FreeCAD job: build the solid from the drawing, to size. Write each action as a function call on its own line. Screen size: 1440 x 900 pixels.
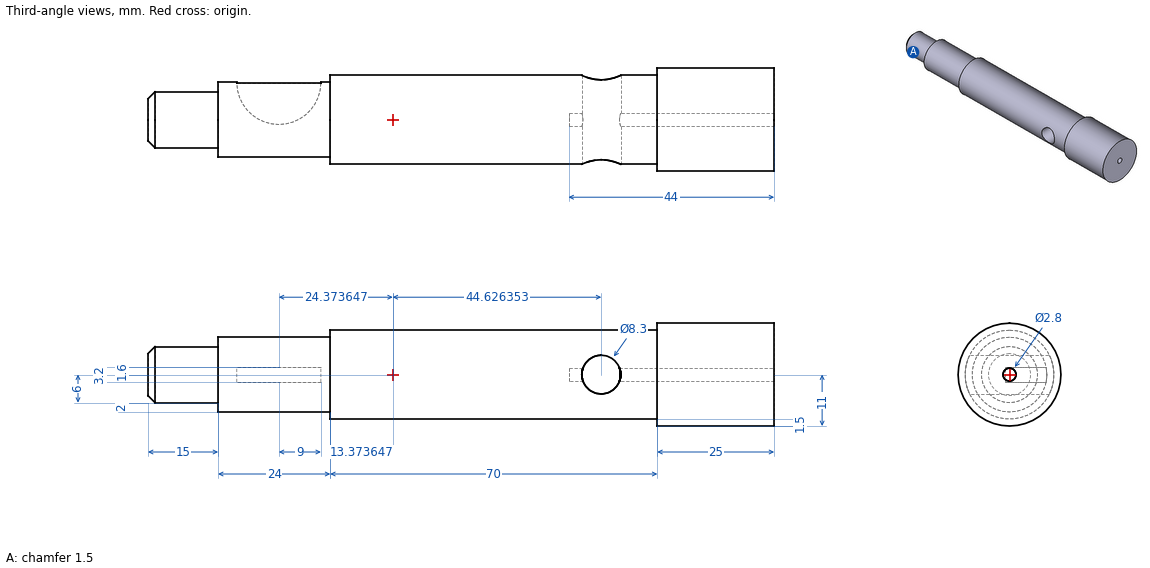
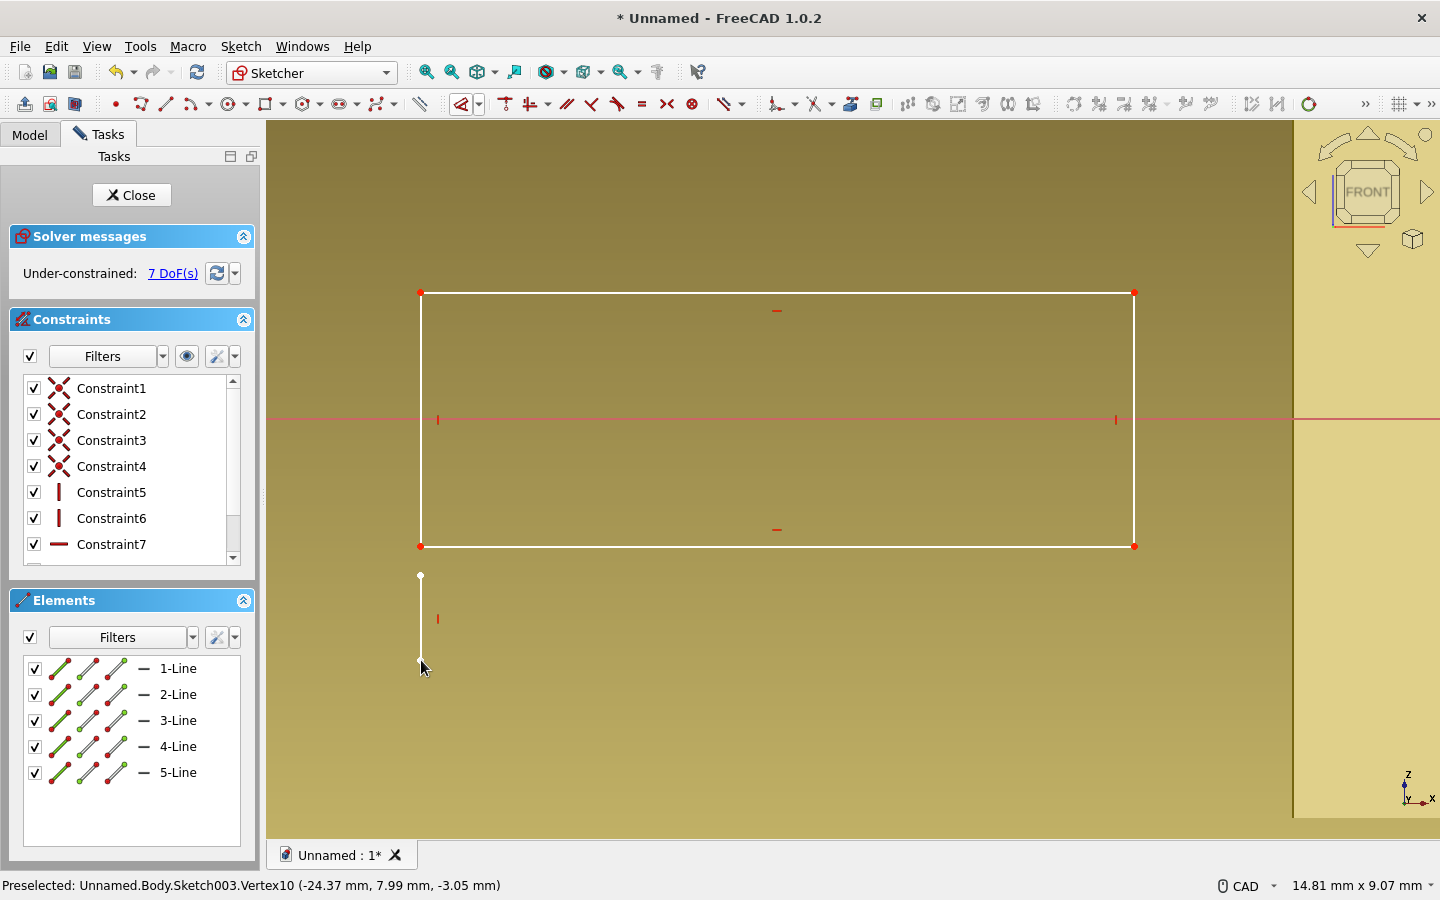
click(421, 601)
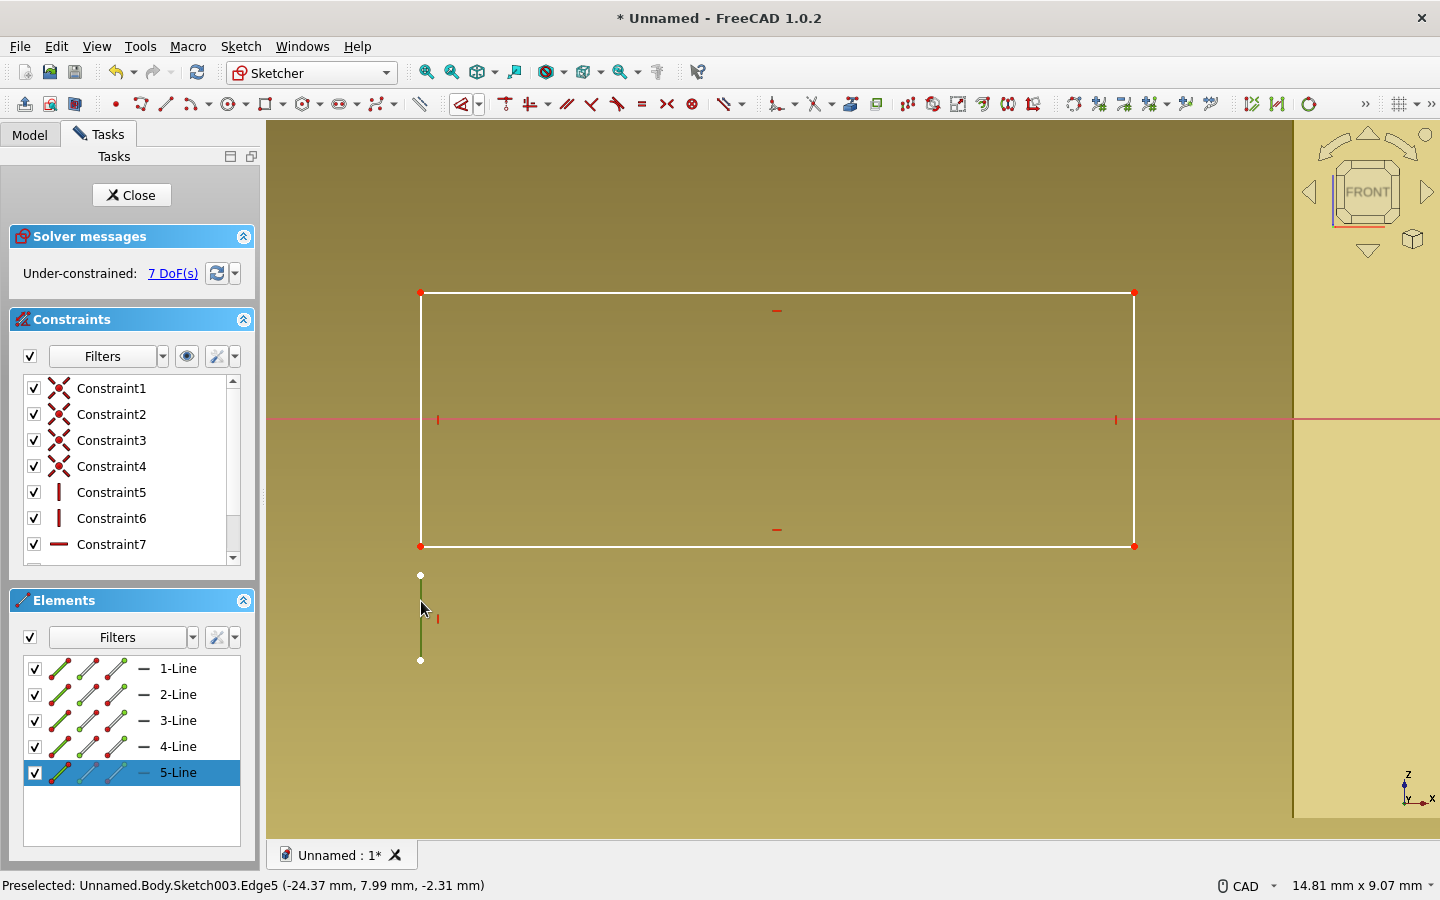
click(420, 104)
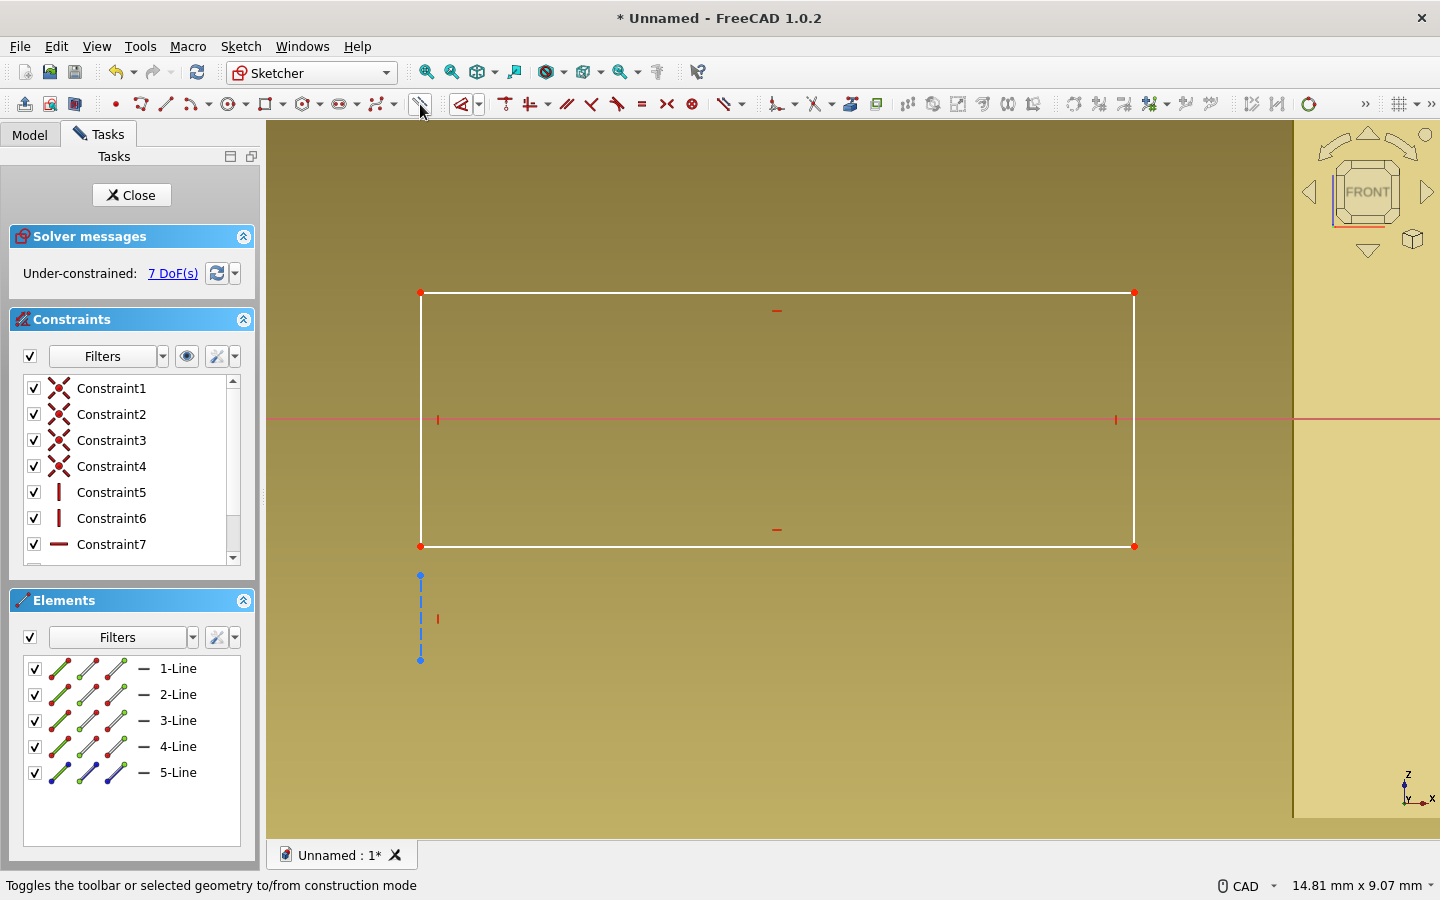
click(635, 547)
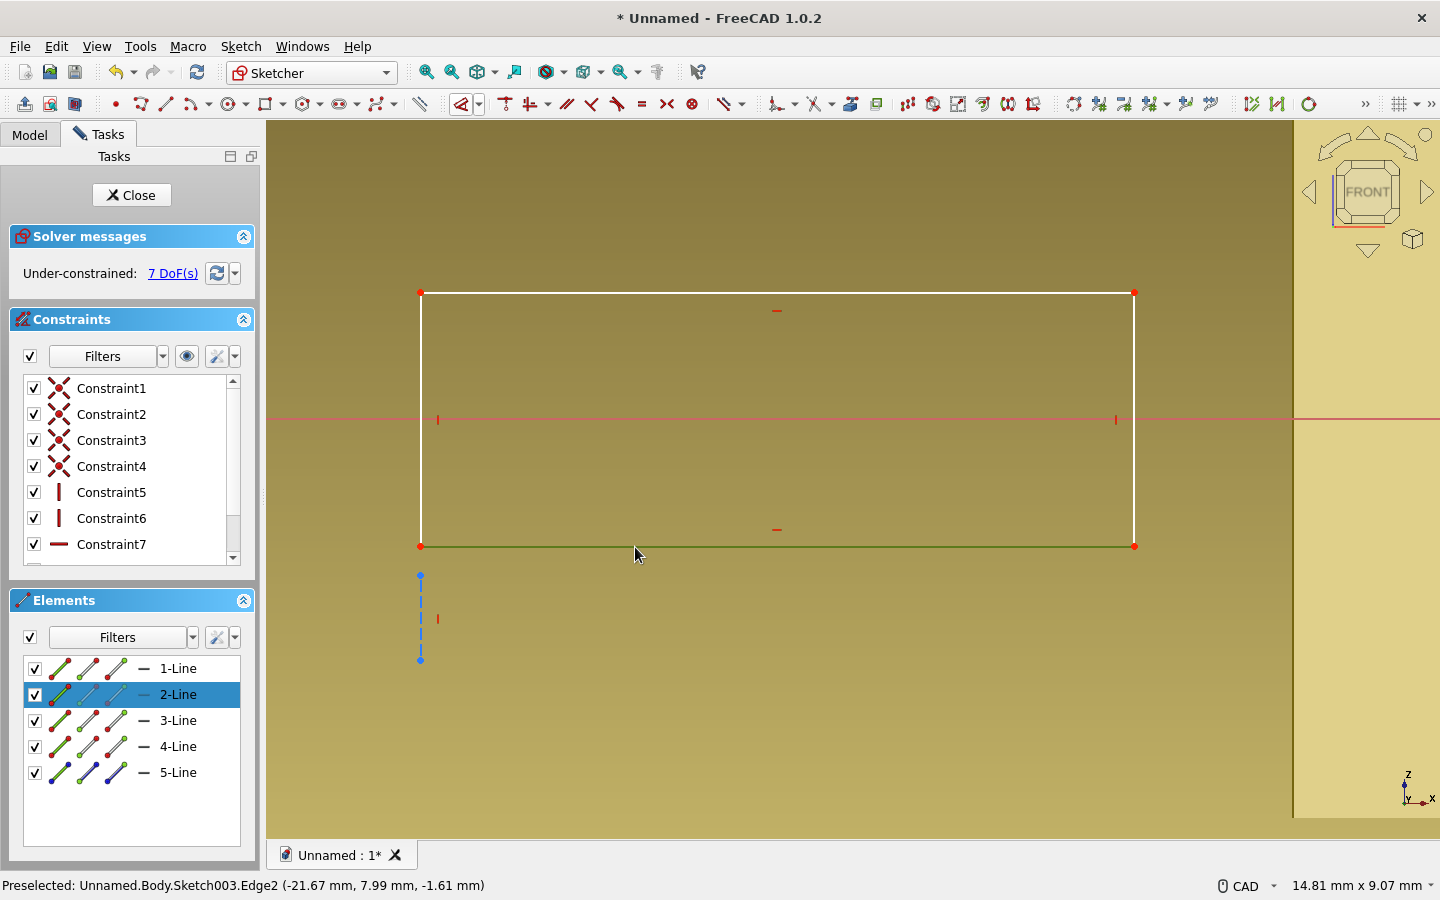
key(l)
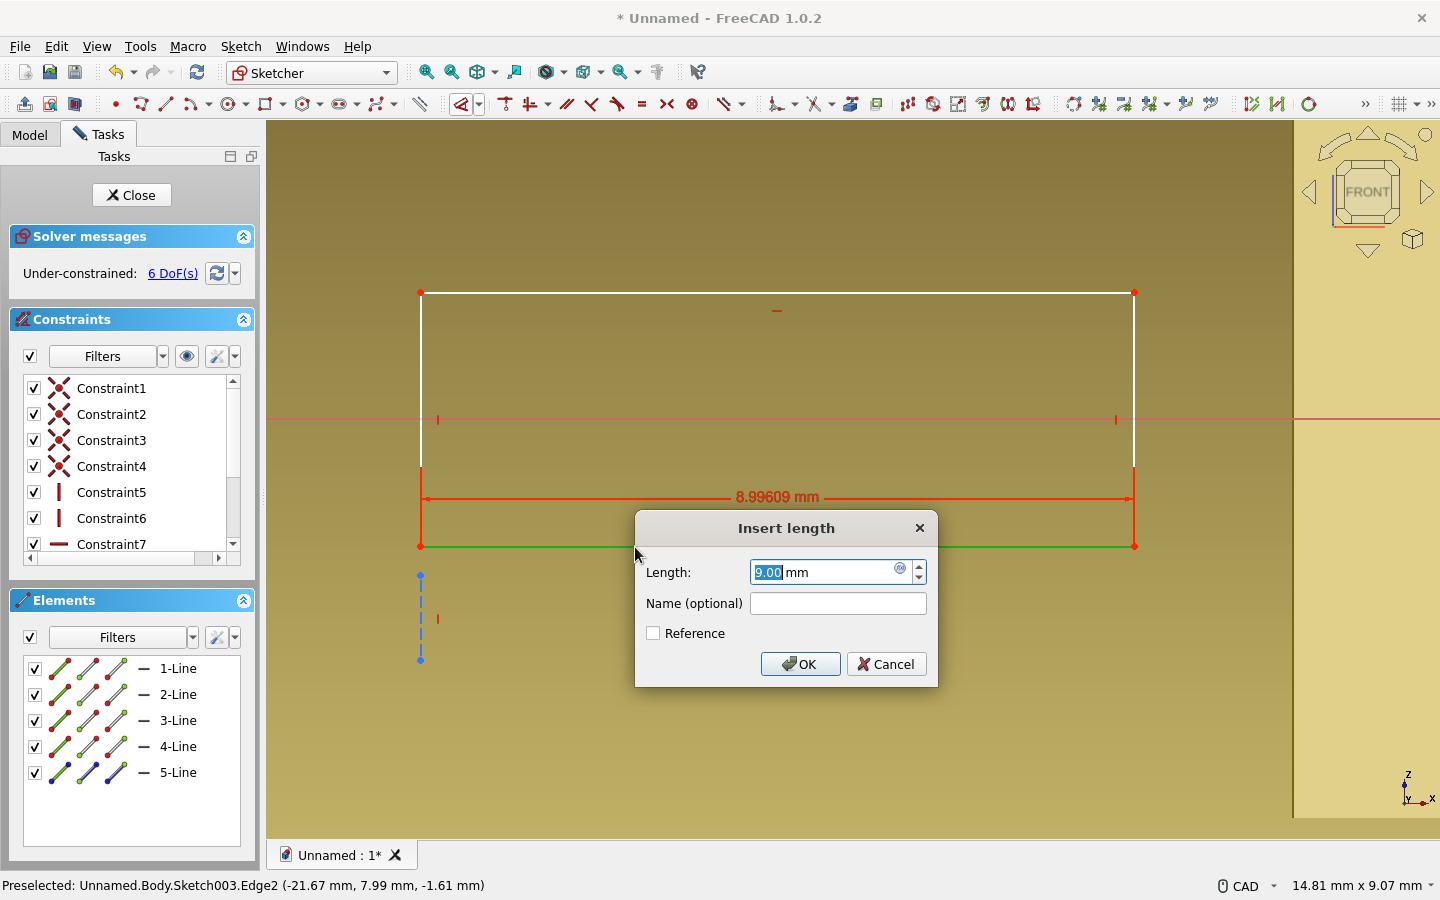
text(9)
key(Return)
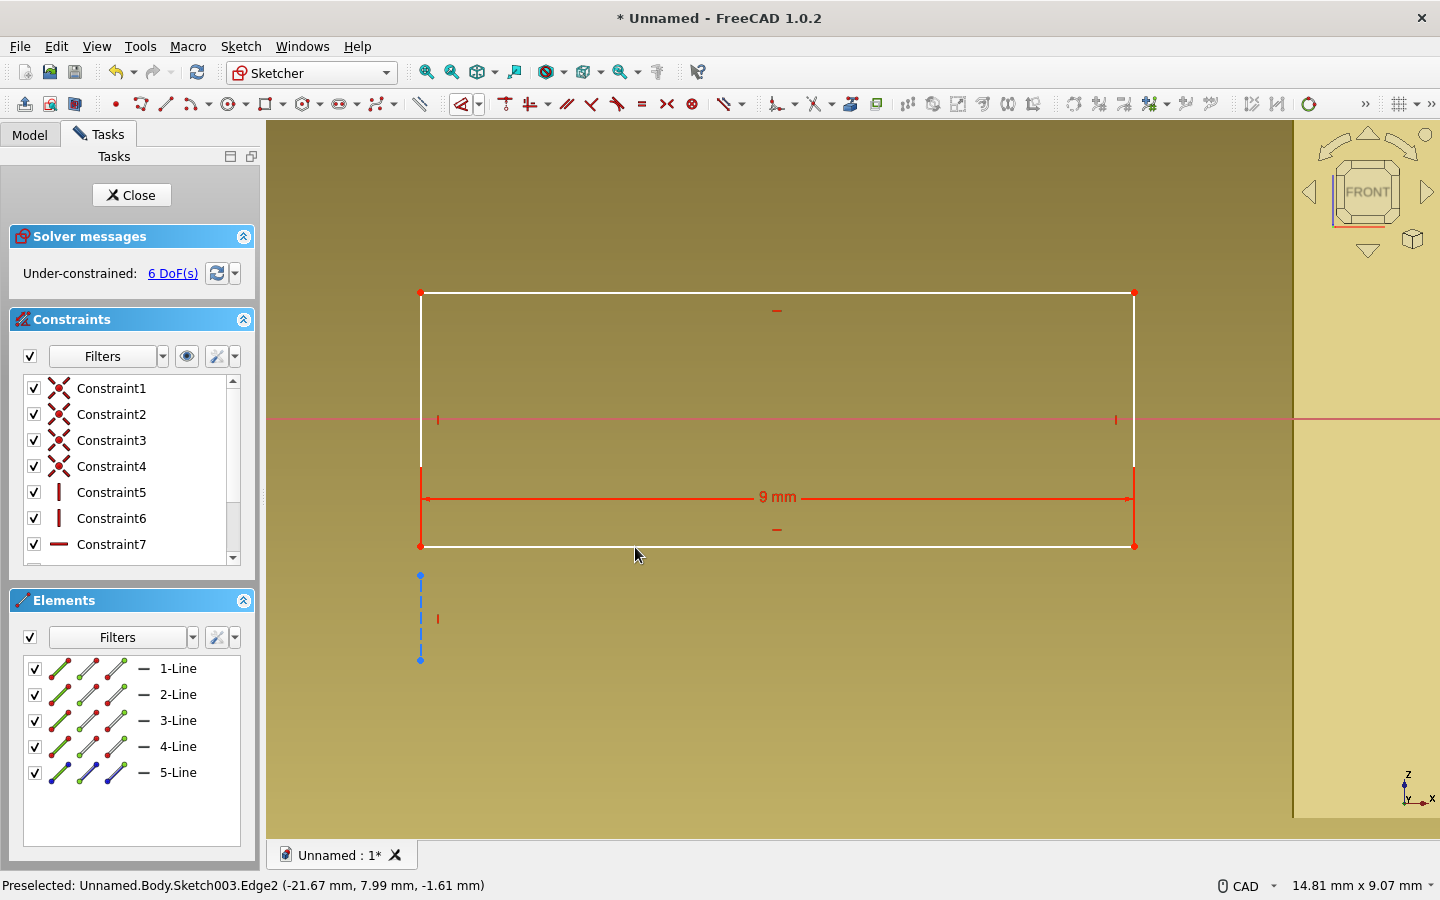
click(421, 369)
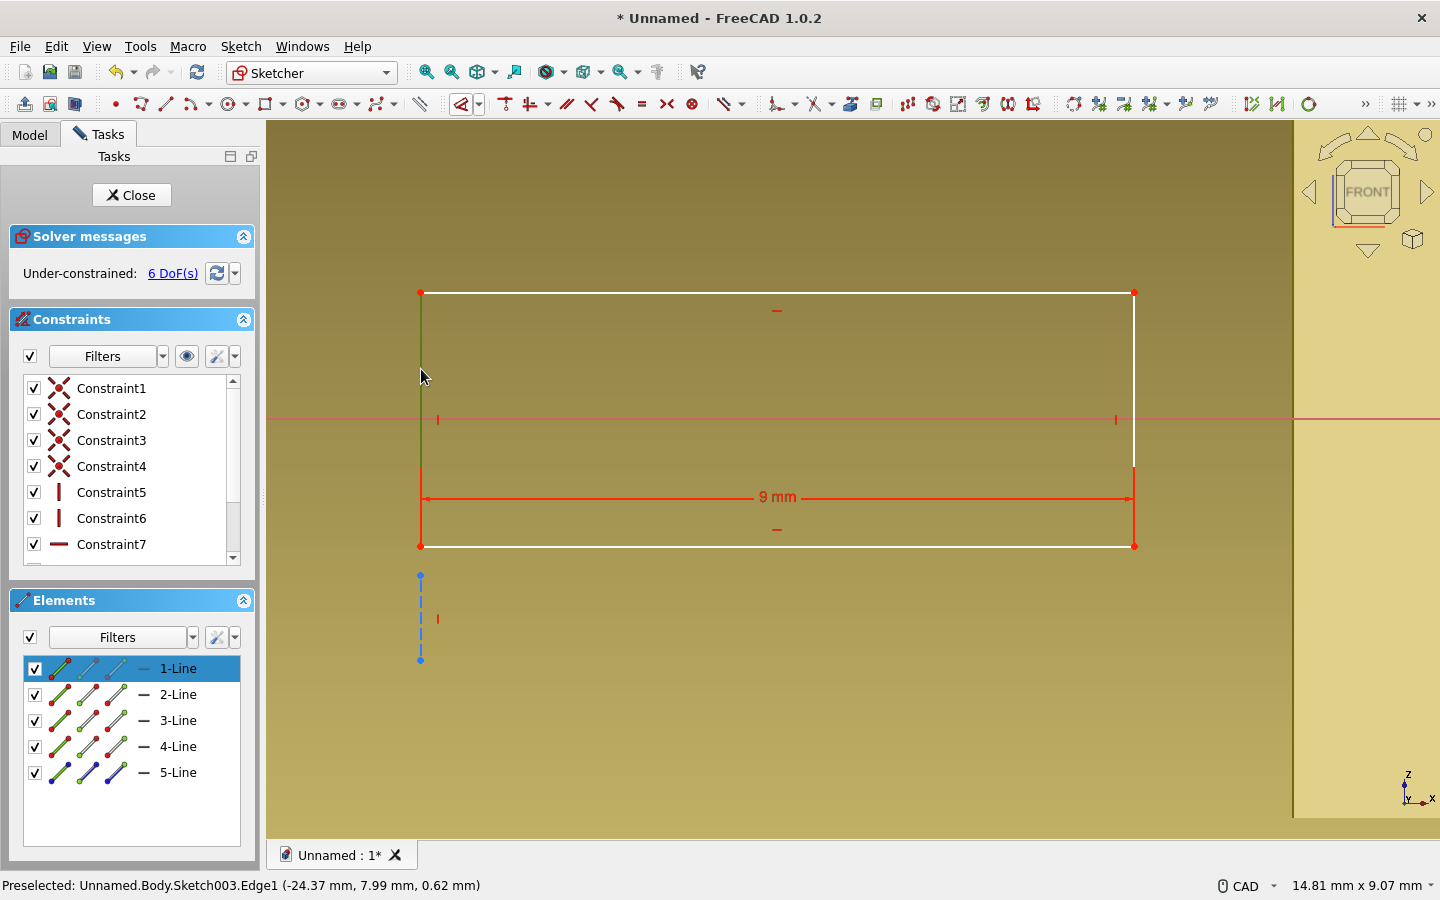
key(i)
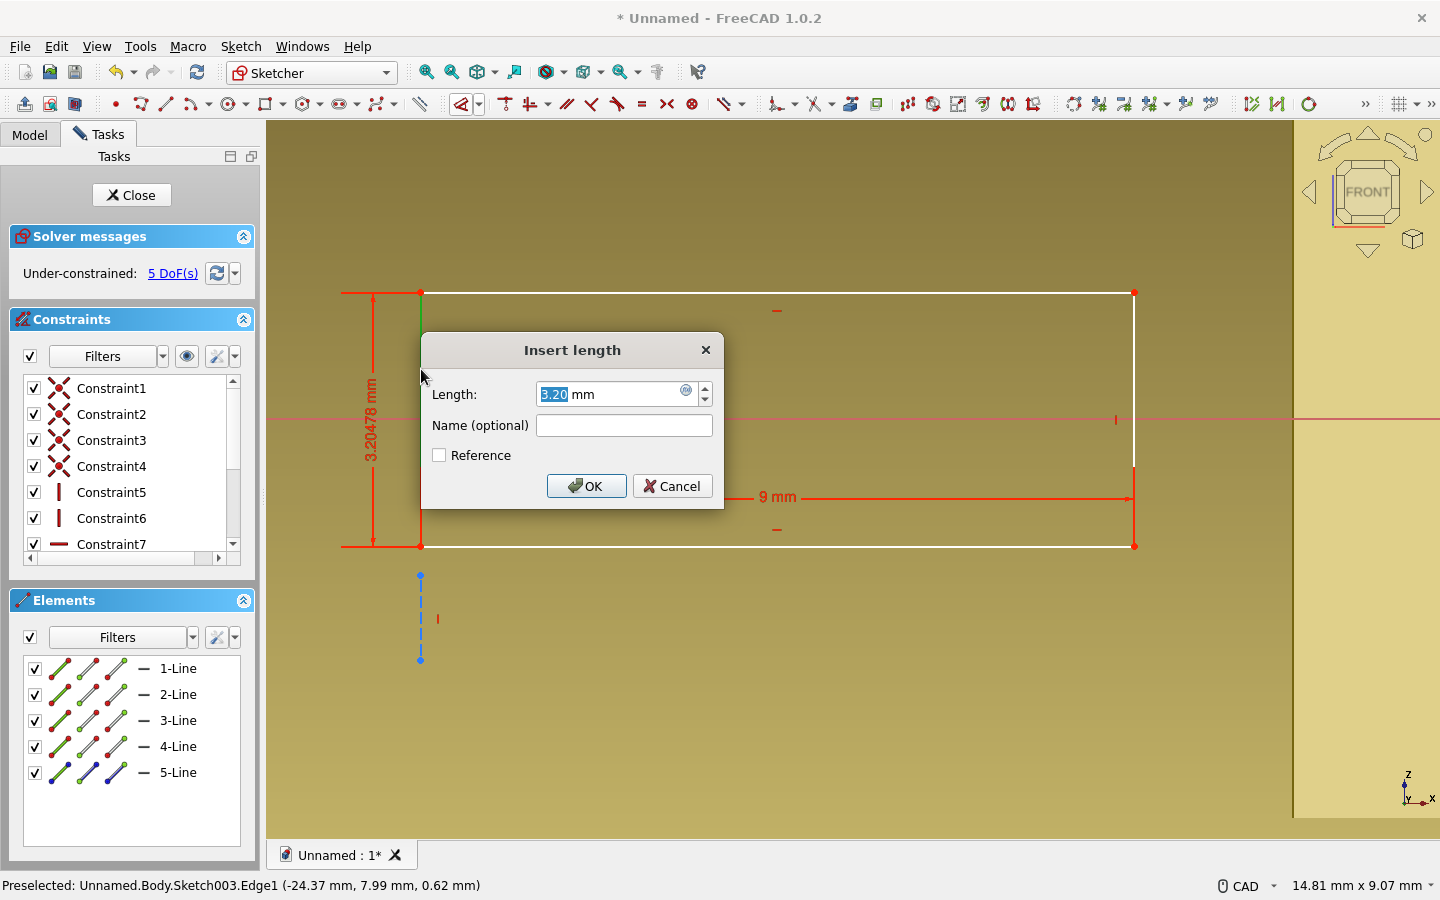
text(3.2)
key(Return)